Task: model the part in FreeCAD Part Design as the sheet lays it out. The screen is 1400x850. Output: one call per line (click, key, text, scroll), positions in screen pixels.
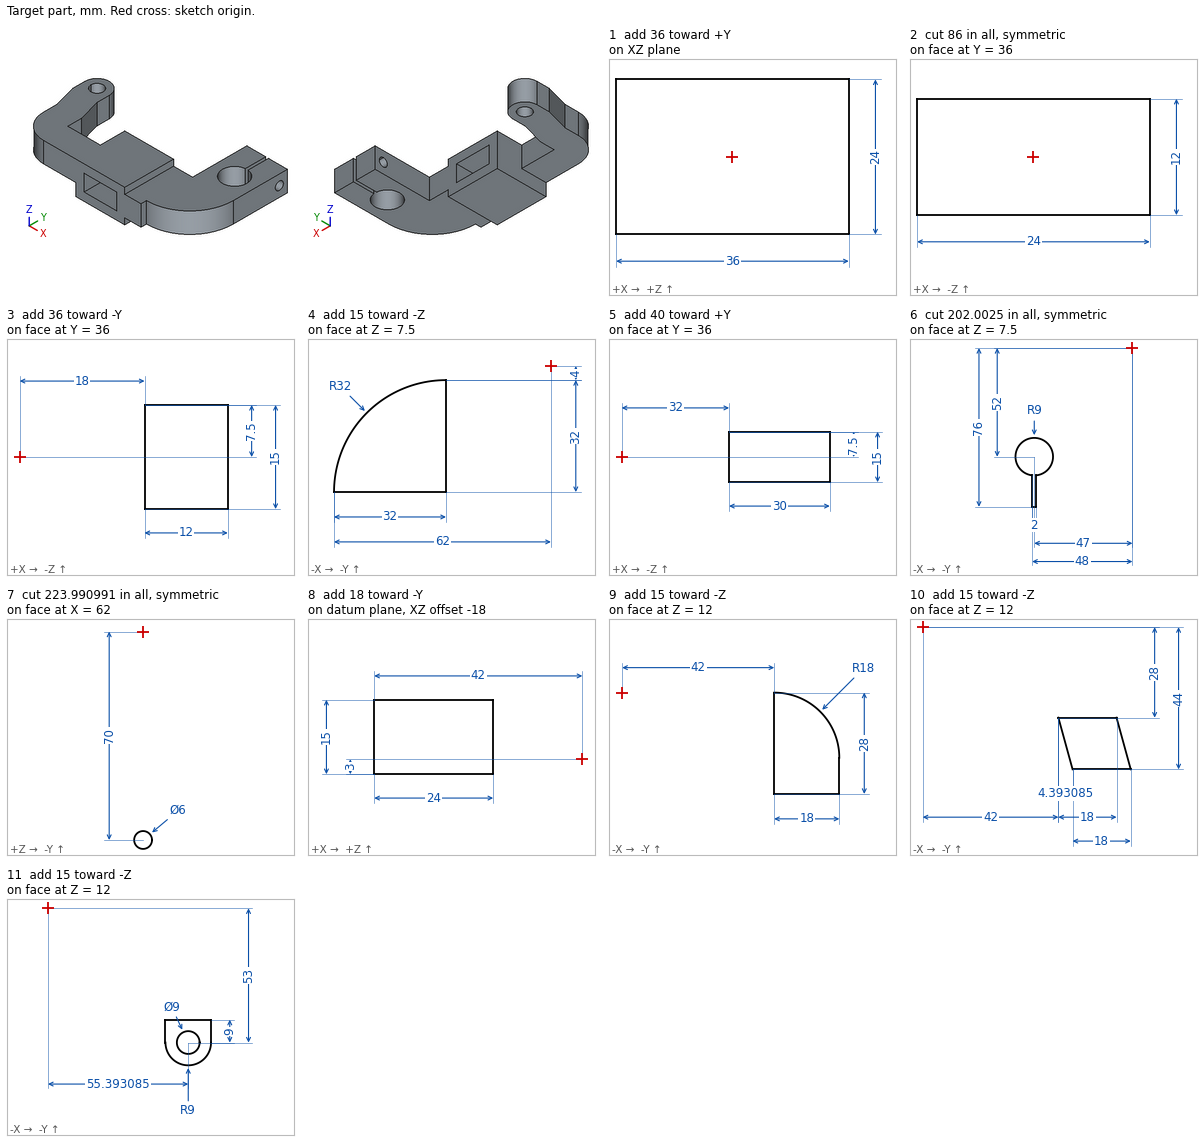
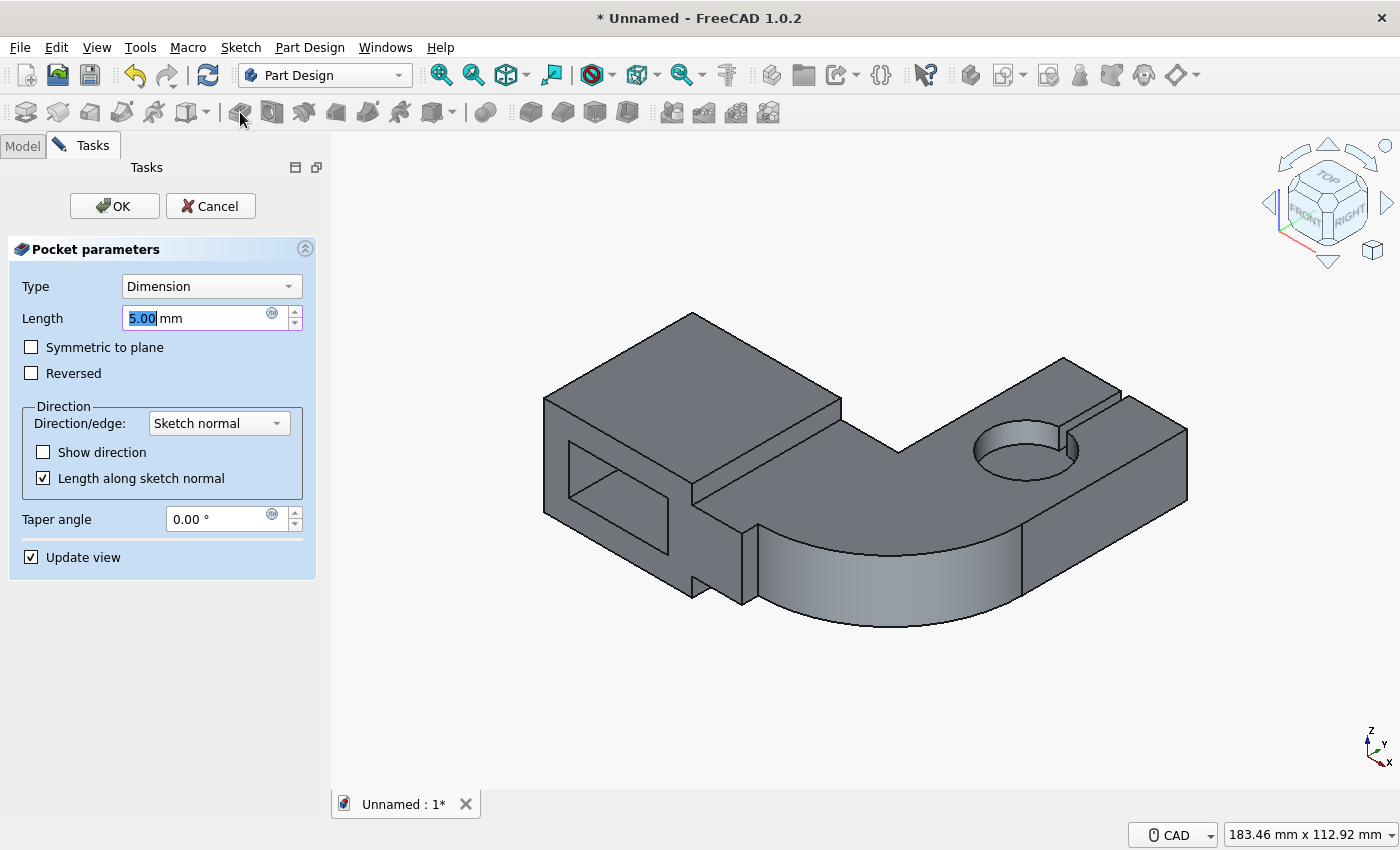
text(202.0025)
key(Tab)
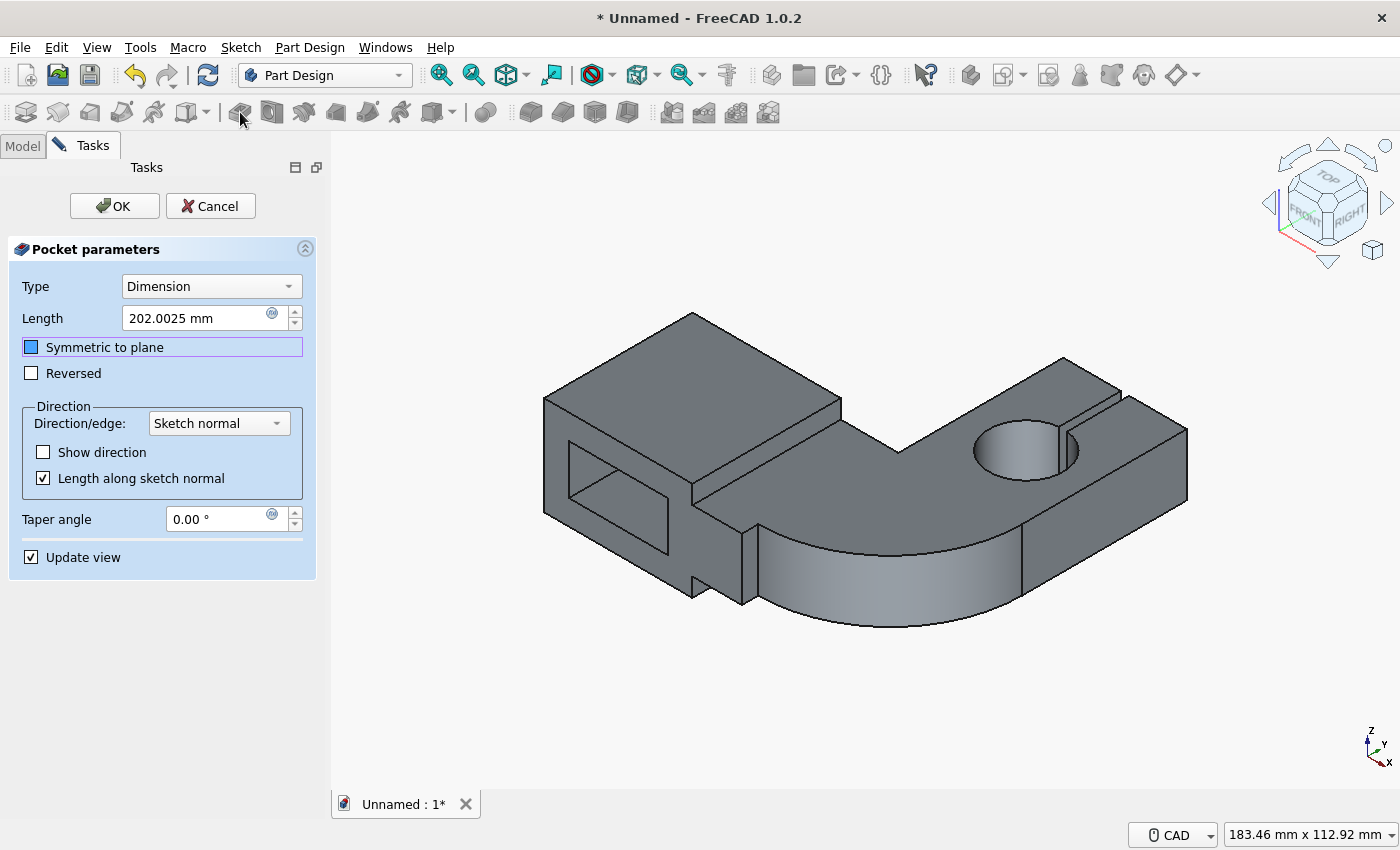
click(30, 347)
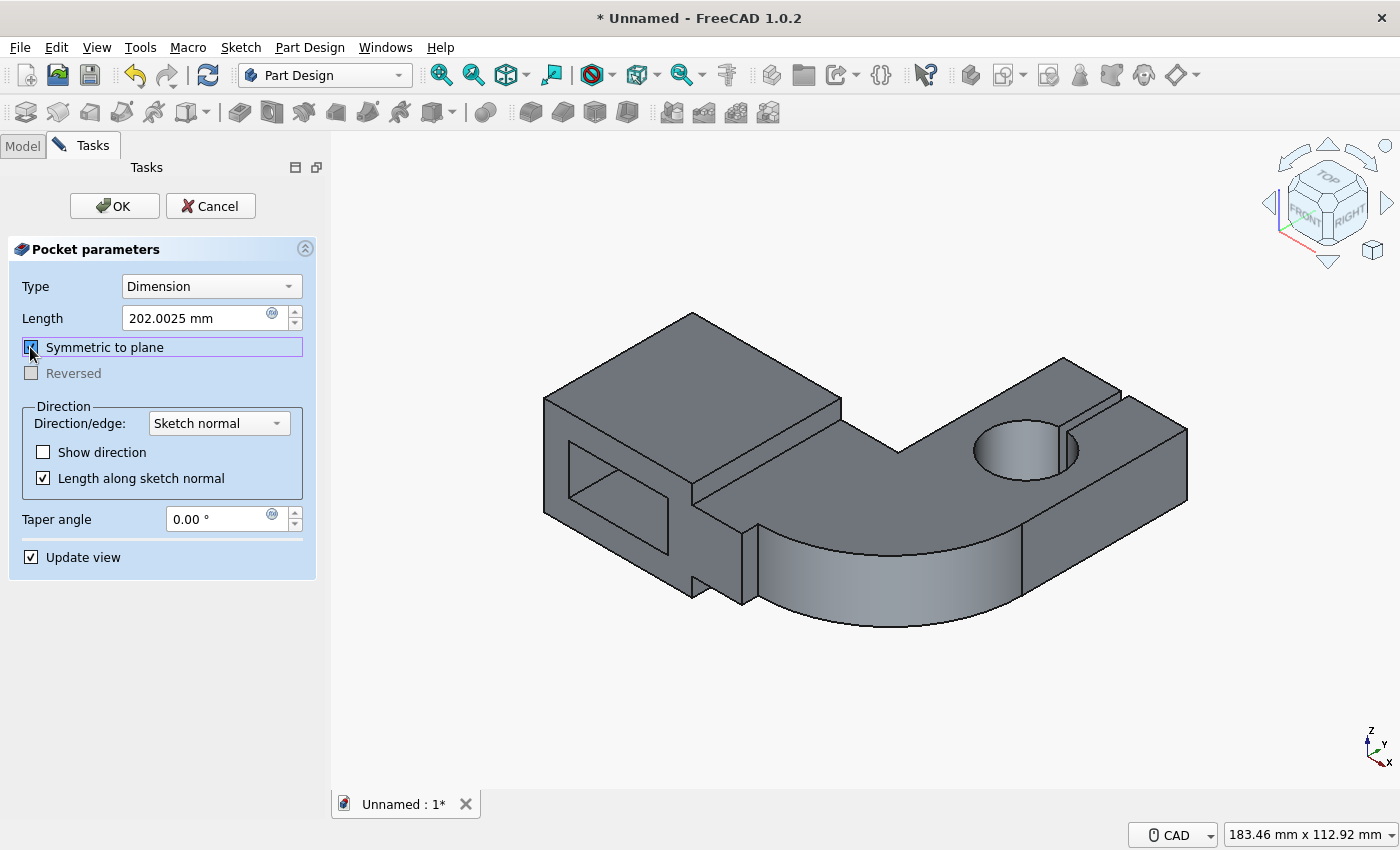
click(115, 206)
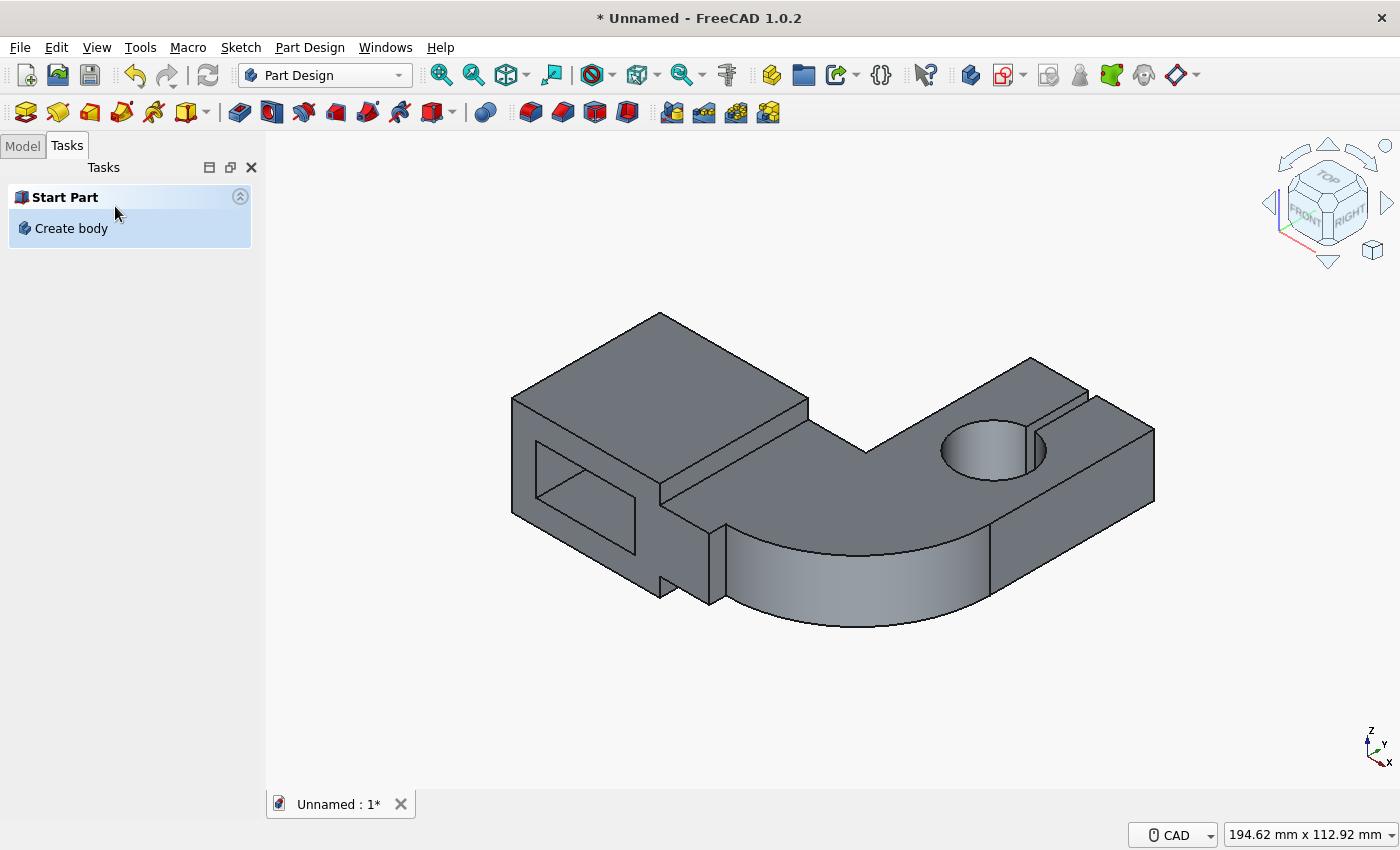
click(1119, 484)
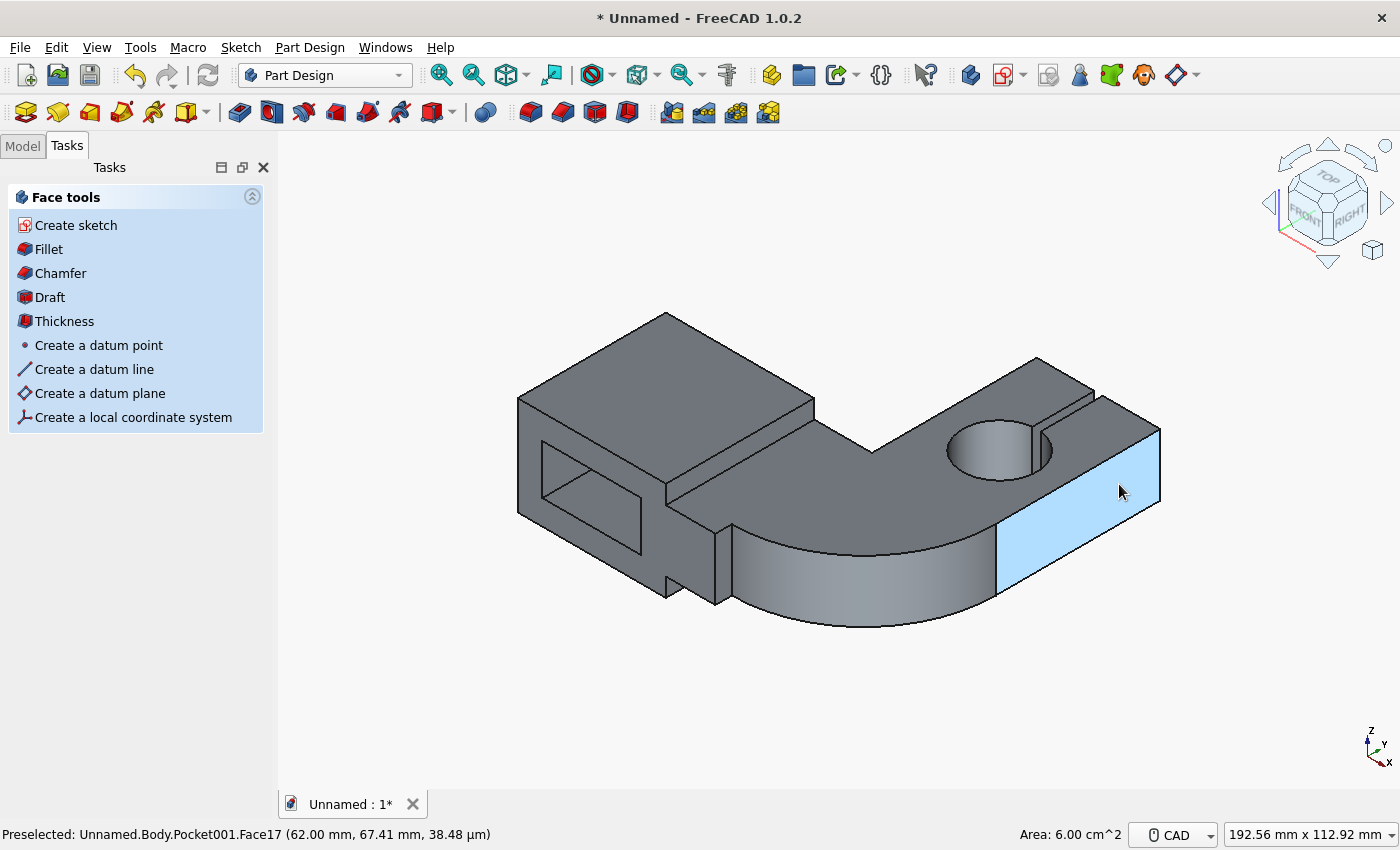
click(1004, 76)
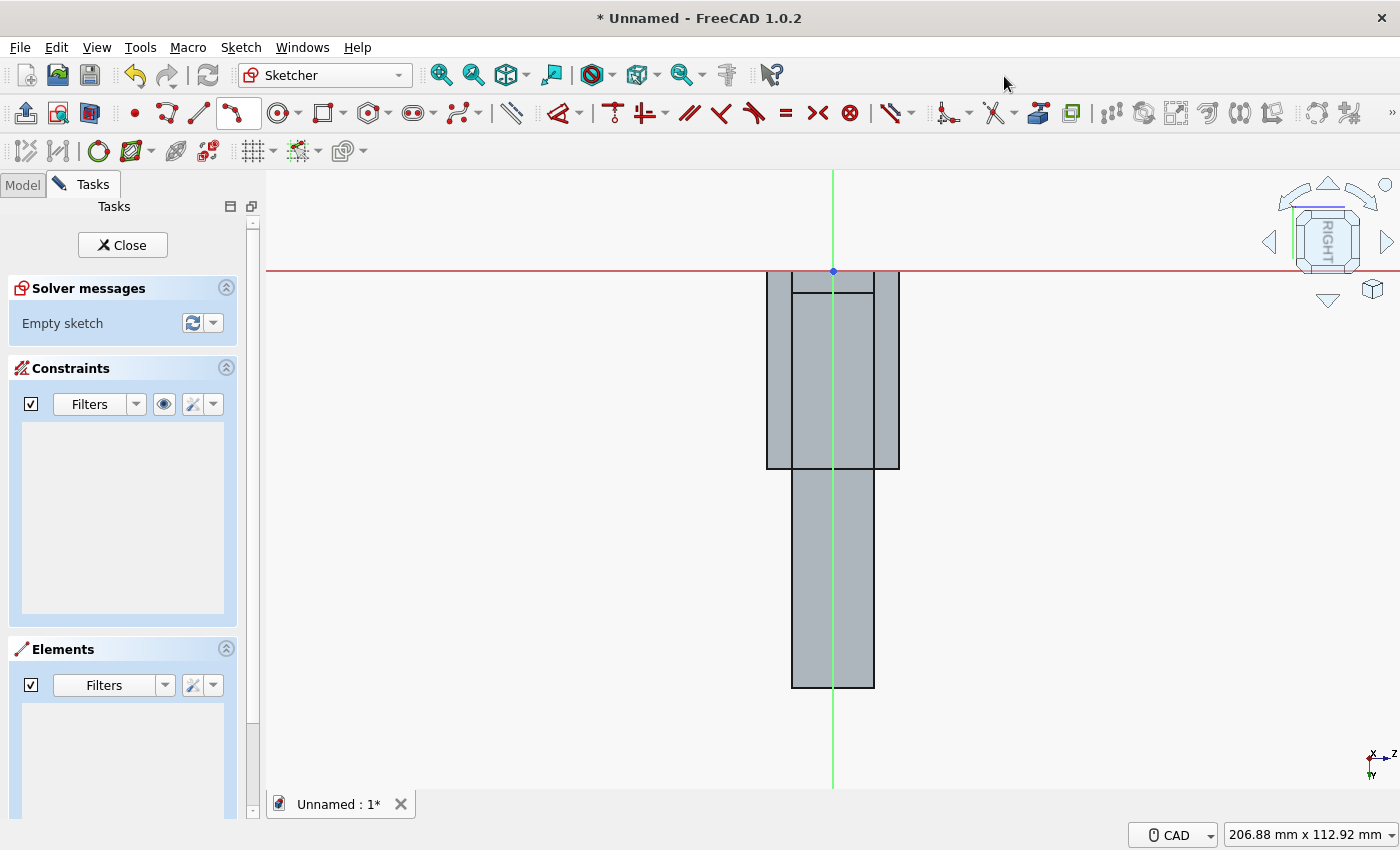
scroll(840, 672, up, 12)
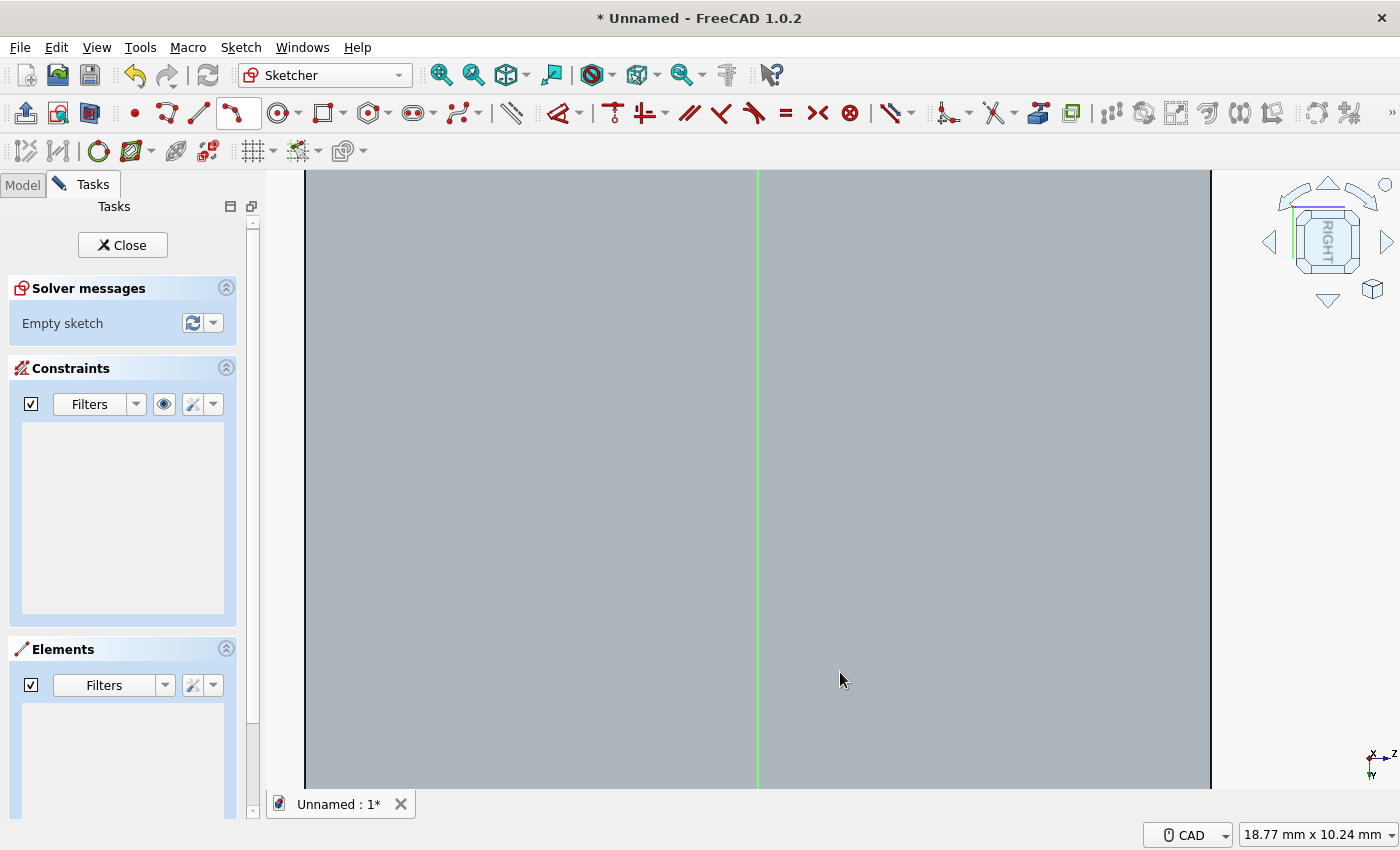
key(g)
key(c)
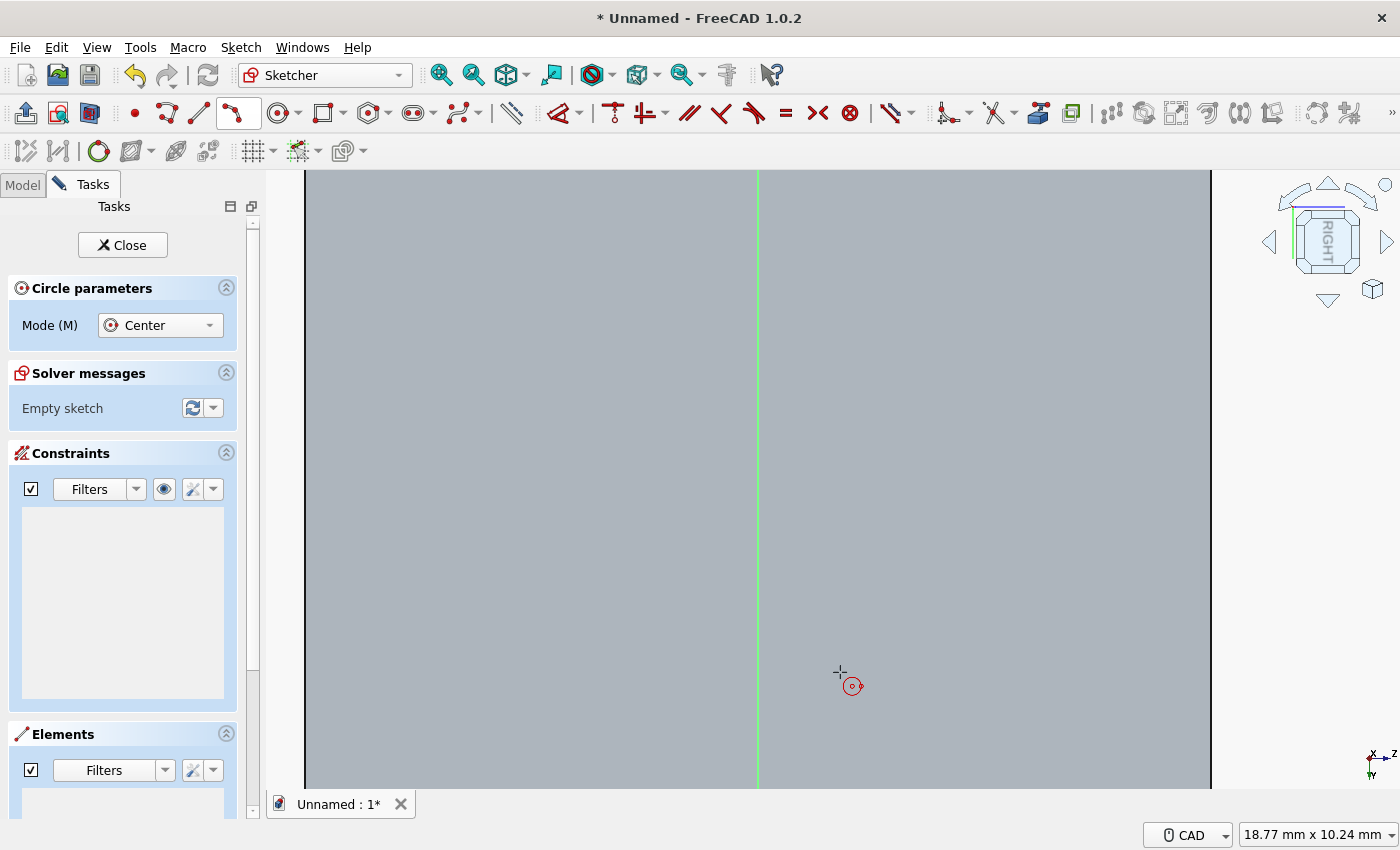
click(758, 475)
click(886, 347)
key(Escape)